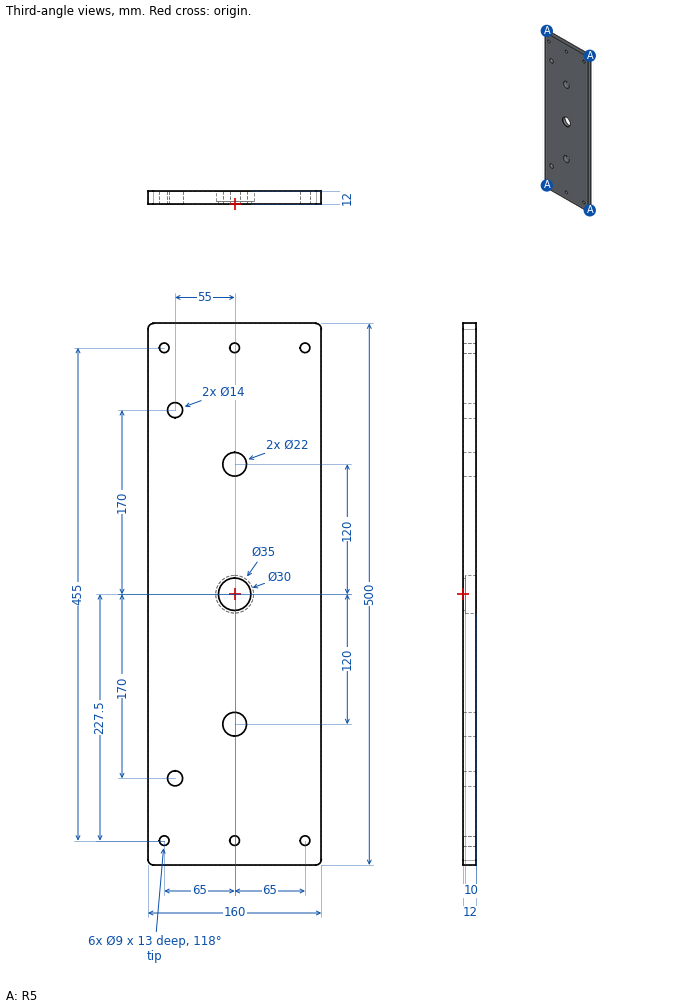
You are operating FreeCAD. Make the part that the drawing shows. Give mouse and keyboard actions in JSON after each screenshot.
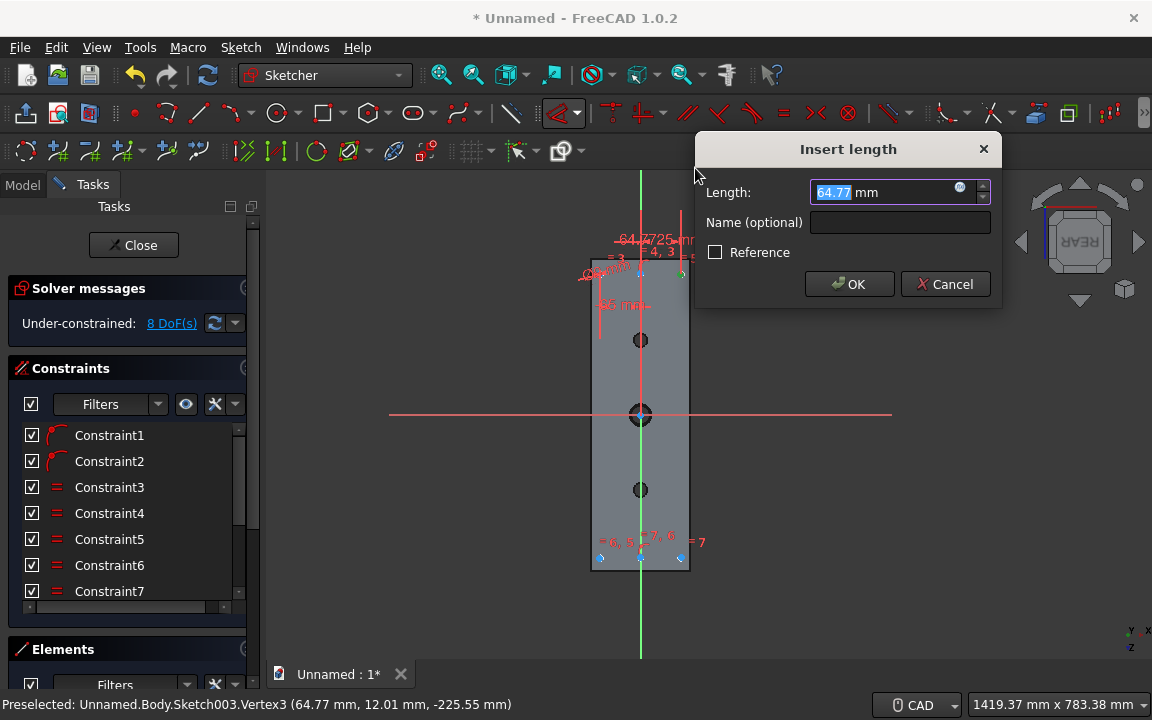
{"action": "type", "text": "65"}
{"action": "key", "text": "Return"}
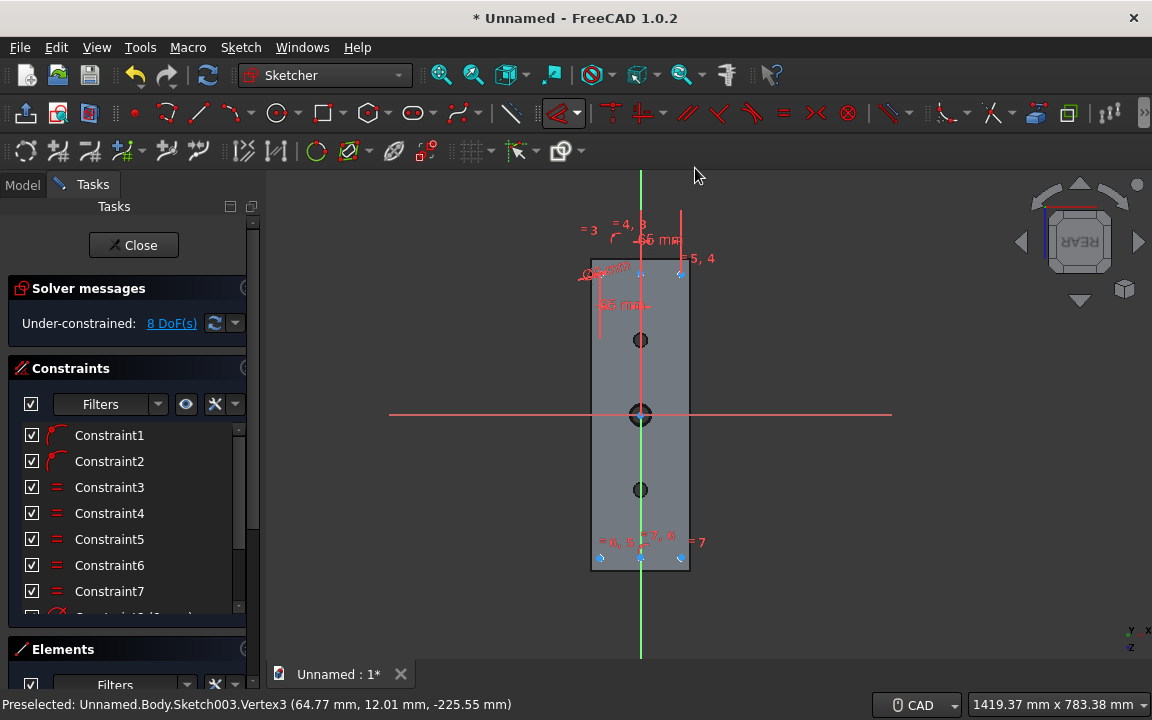
{"action": "left_click", "coordinate": [600, 558]}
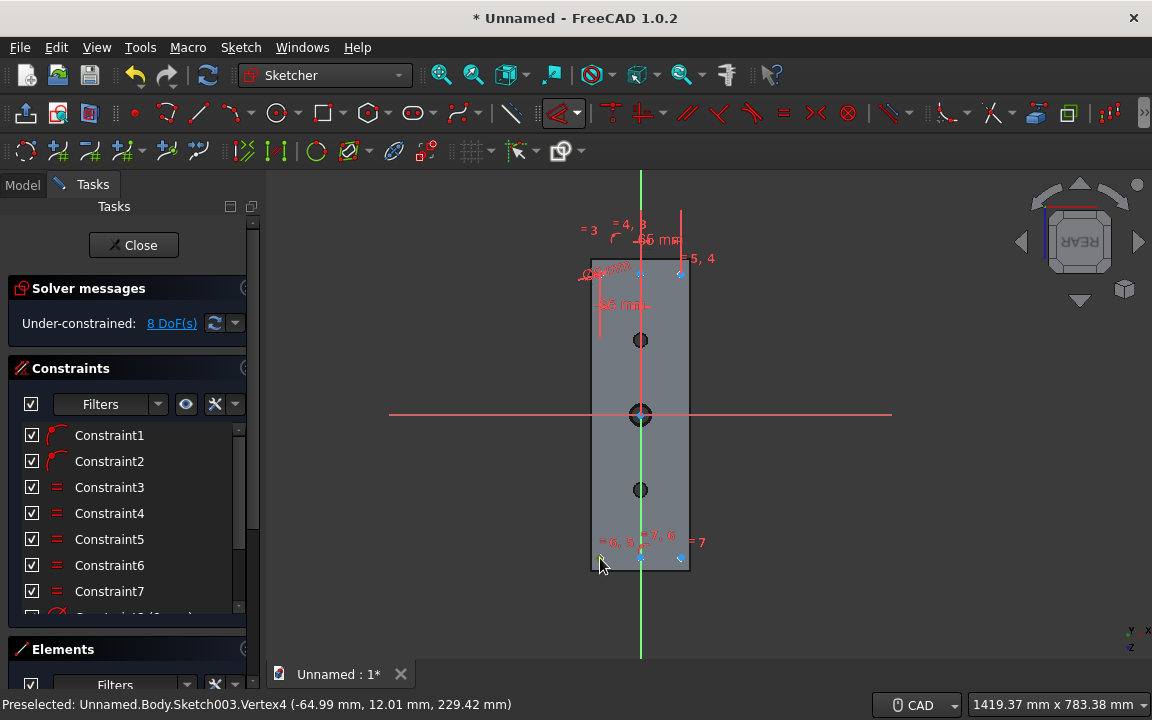
{"action": "left_click", "coordinate": [580, 114]}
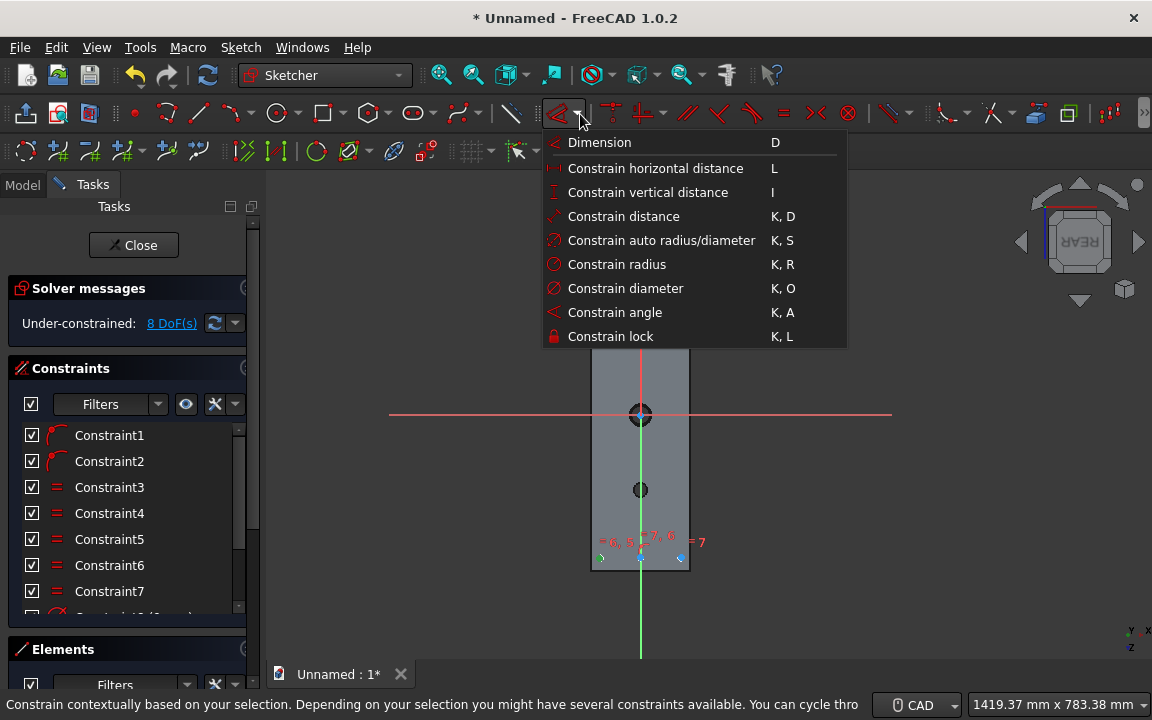
{"action": "left_click", "coordinate": [695, 168]}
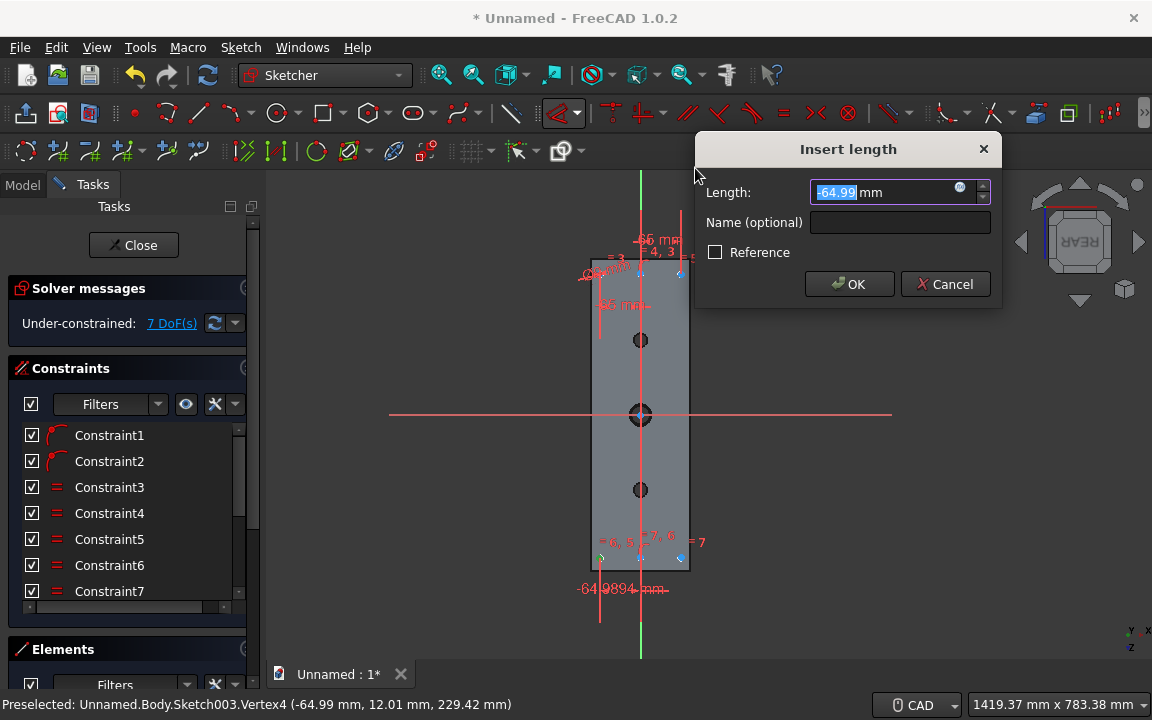
{"action": "type", "text": "-65"}
{"action": "key", "text": "Return"}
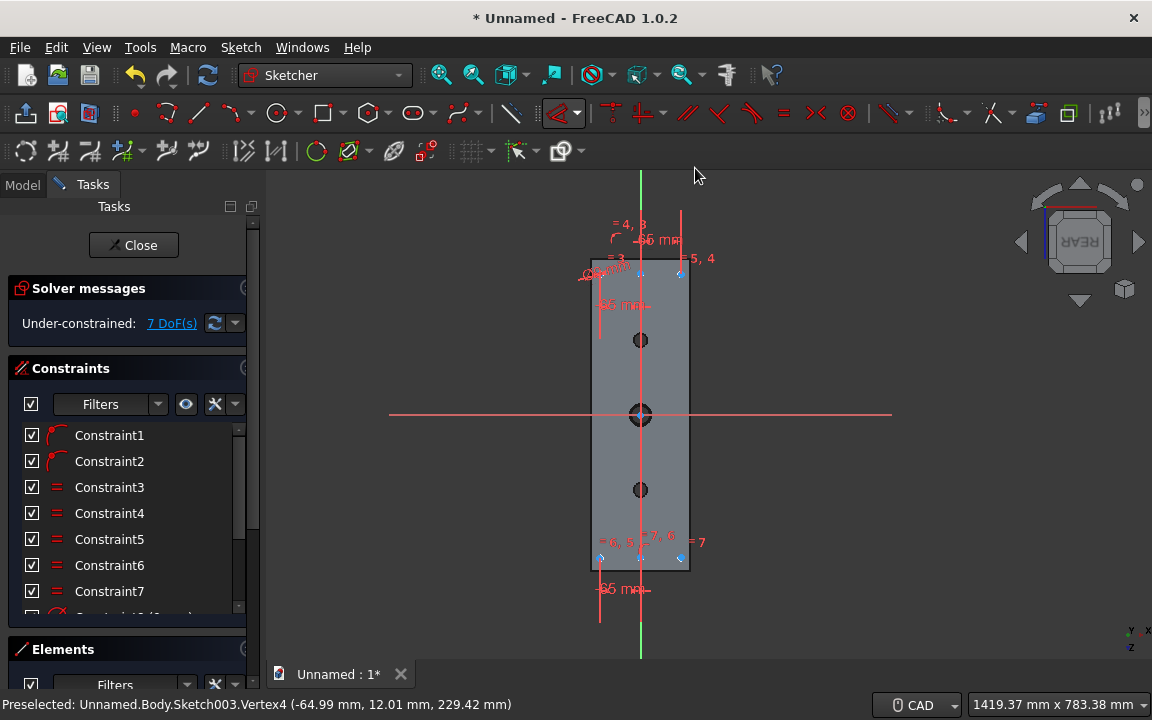
{"action": "left_click", "coordinate": [681, 558]}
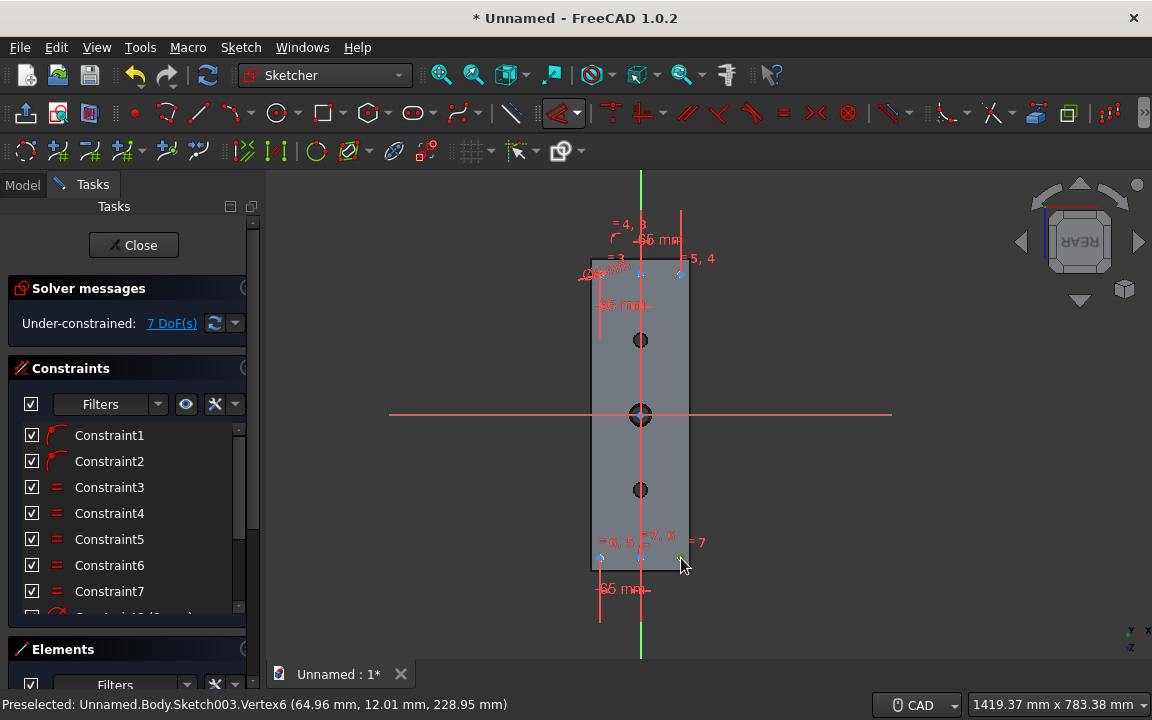
{"action": "left_click", "coordinate": [580, 114]}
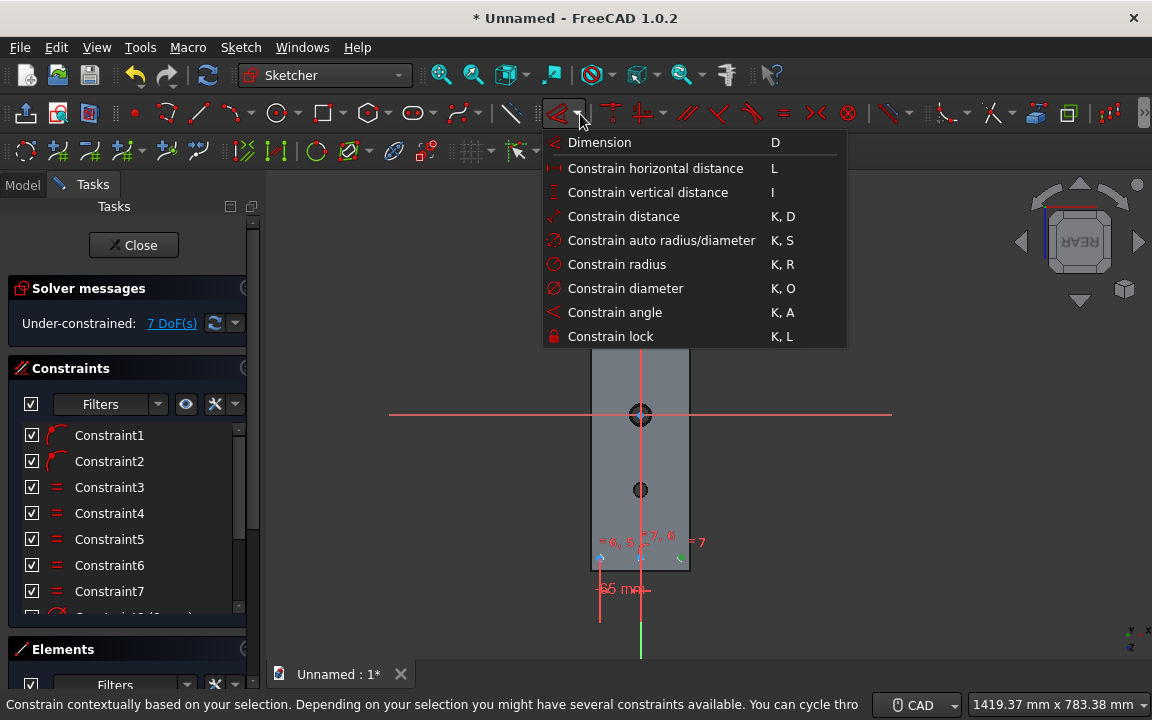
{"action": "left_click", "coordinate": [695, 168]}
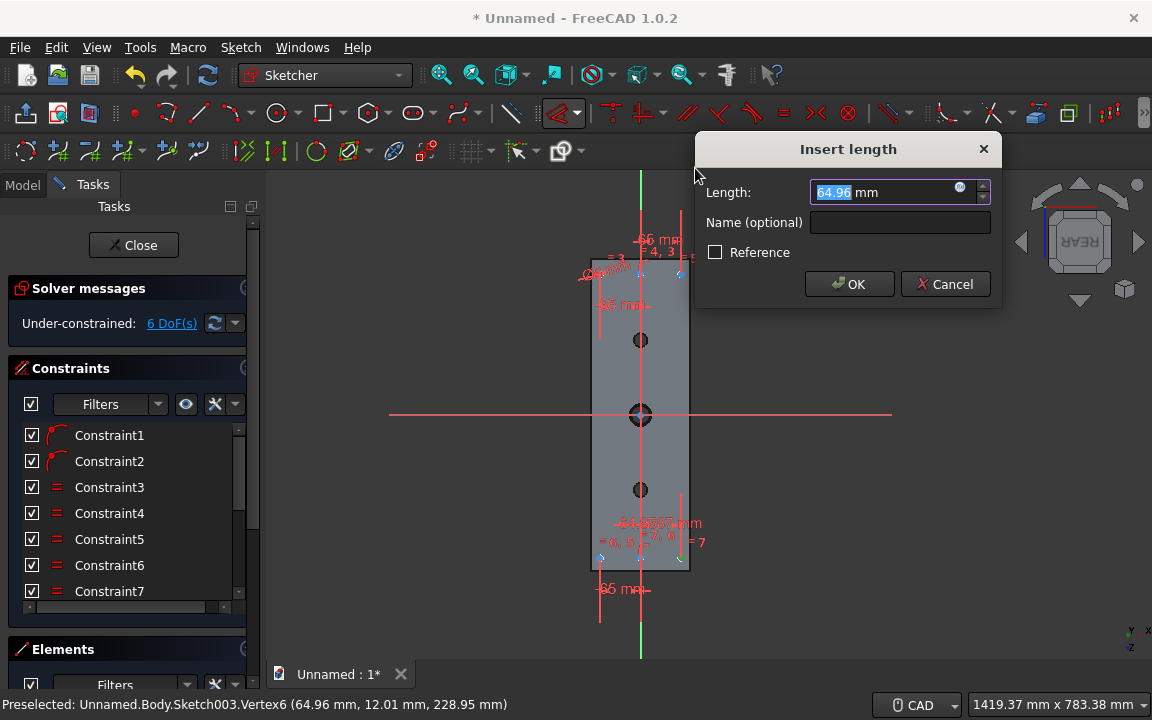
{"action": "type", "text": "65"}
{"action": "key", "text": "Return"}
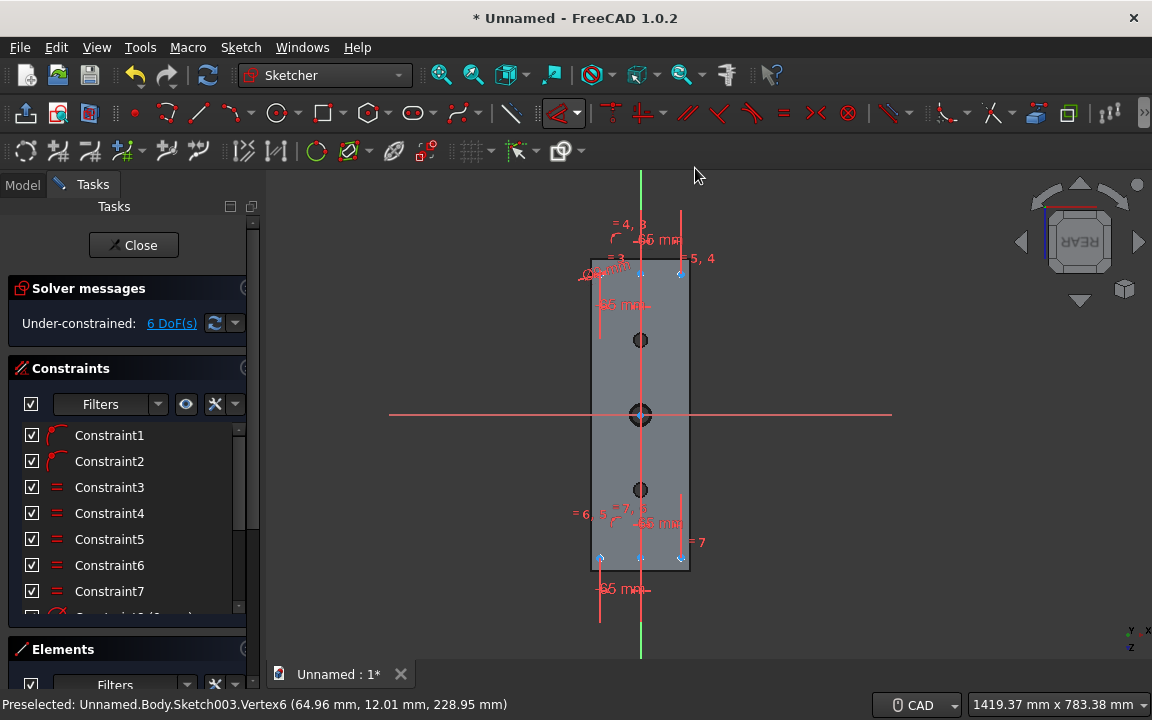
{"action": "left_click", "coordinate": [600, 274]}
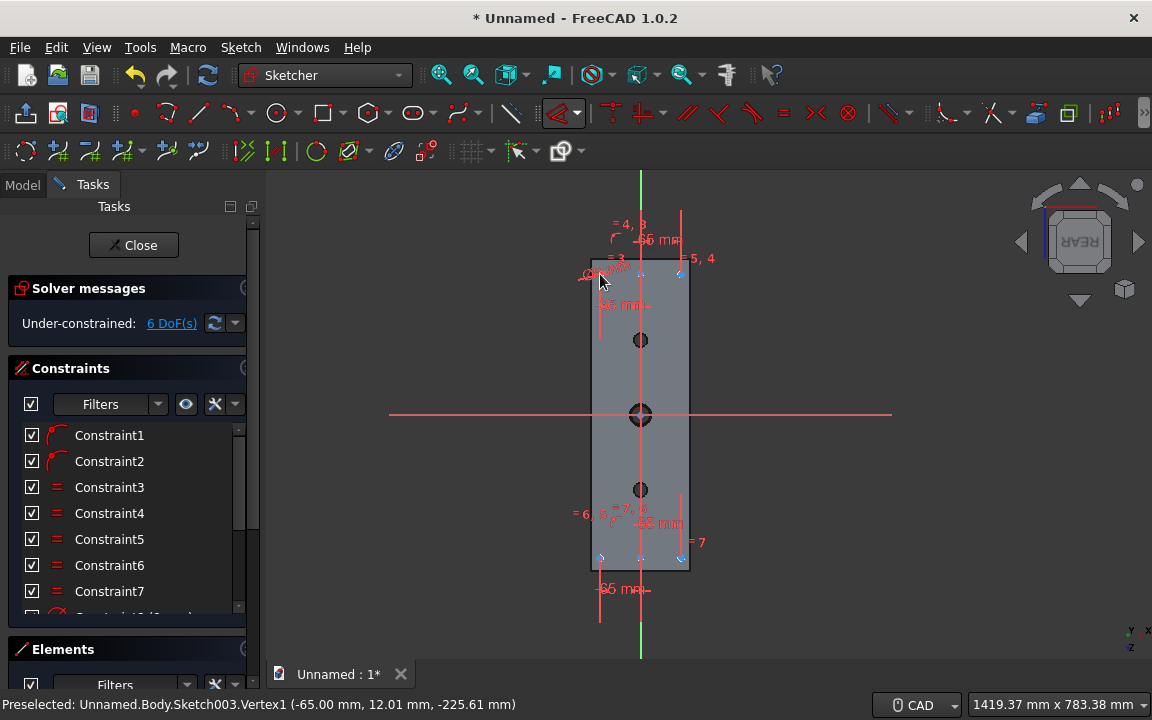
{"action": "left_click", "coordinate": [600, 558]}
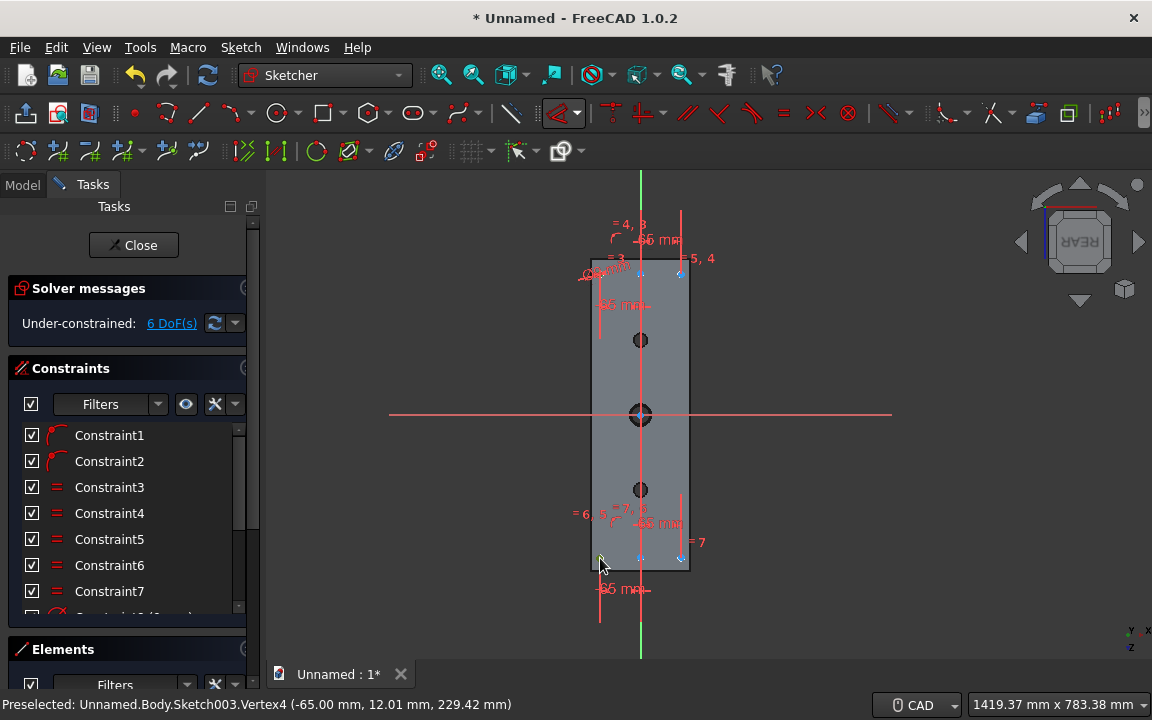
{"action": "left_click", "coordinate": [580, 114]}